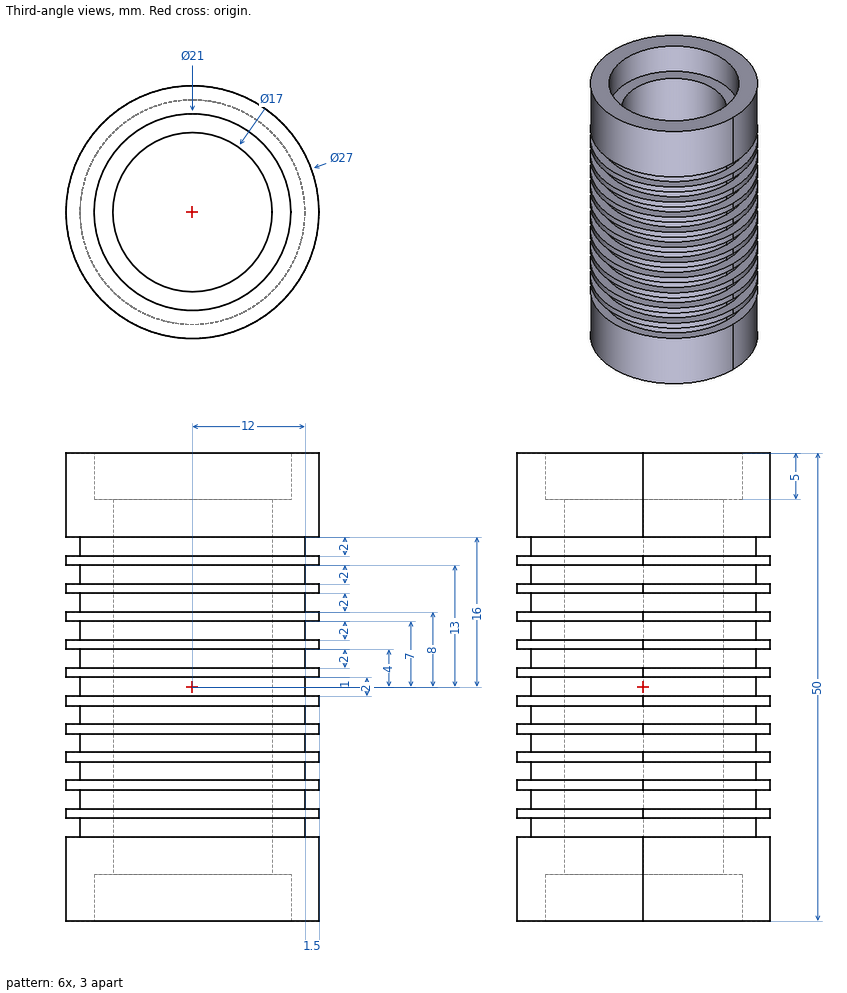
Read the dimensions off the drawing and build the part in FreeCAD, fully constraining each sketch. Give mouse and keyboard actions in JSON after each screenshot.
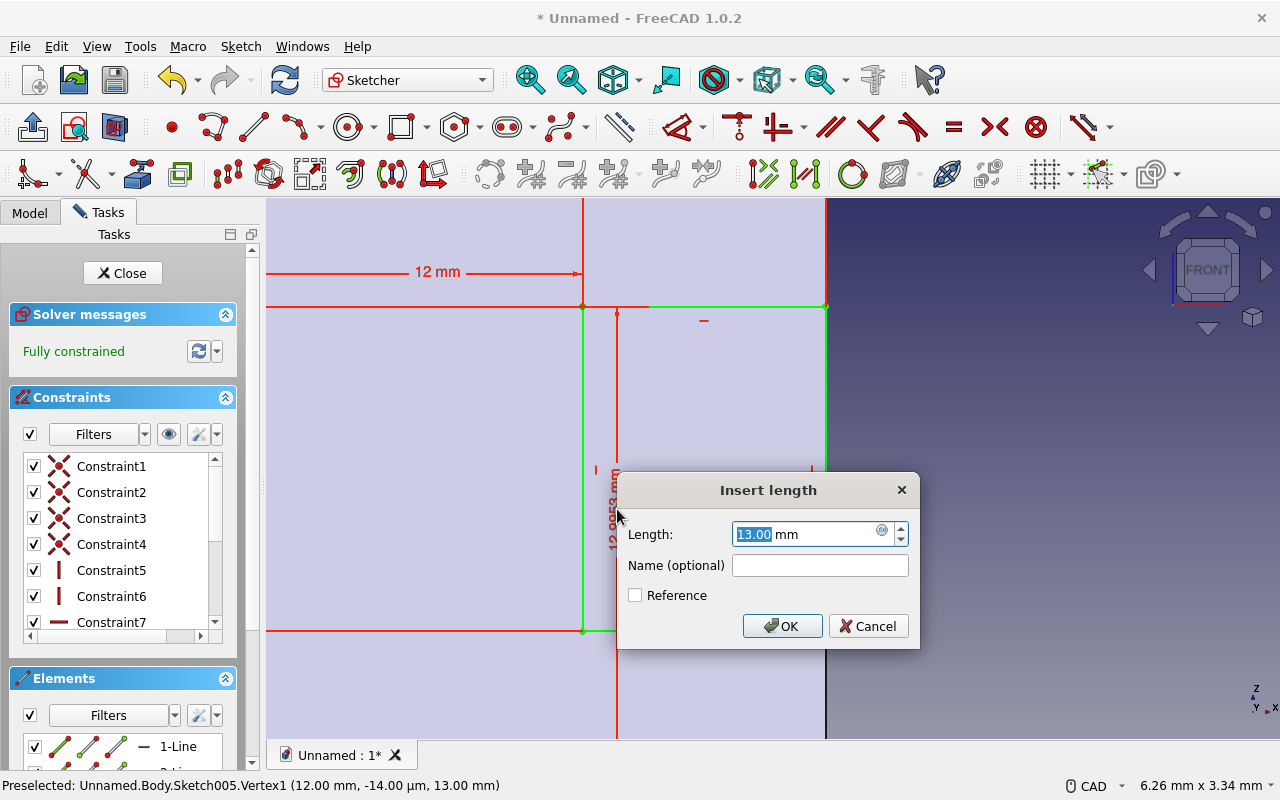
{"action": "type", "text": "13"}
{"action": "key", "text": "Return"}
{"action": "key", "text": "Escape"}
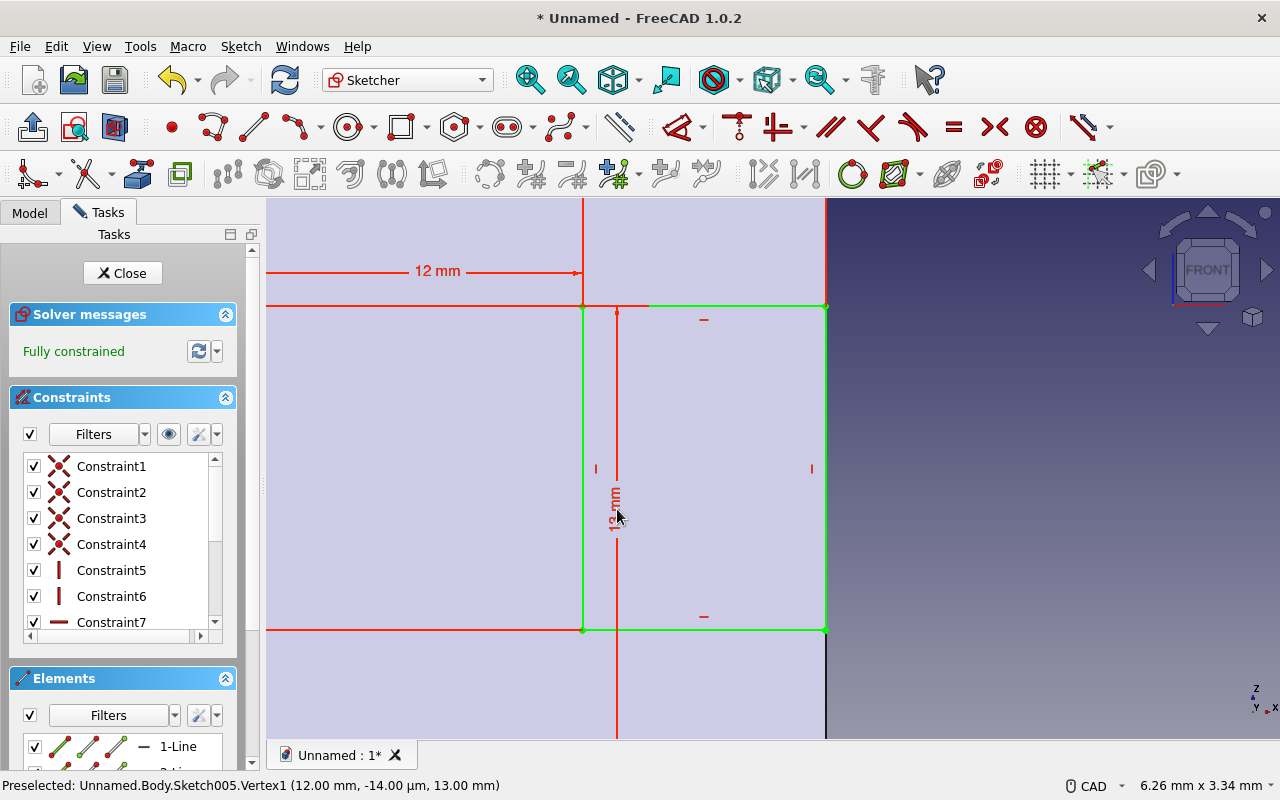
{"action": "left_click", "coordinate": [123, 273]}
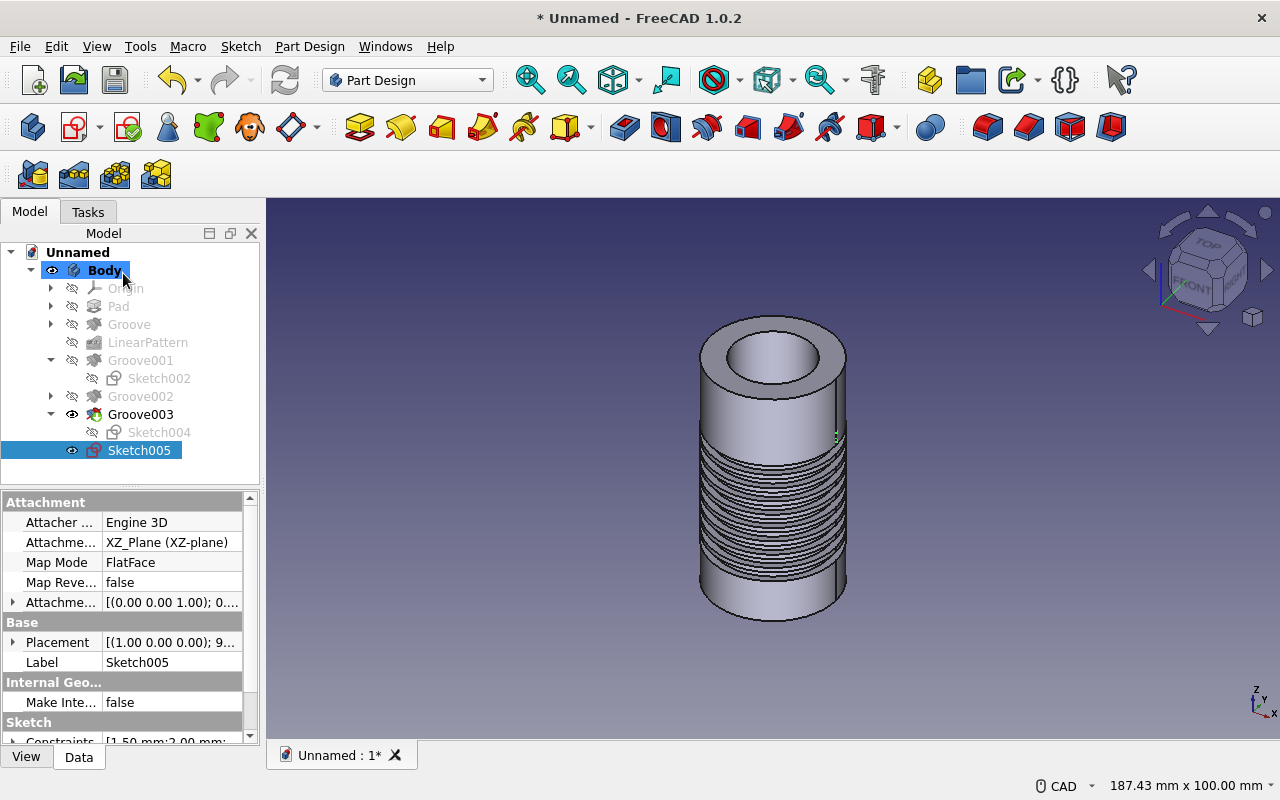
{"action": "left_click", "coordinate": [707, 128]}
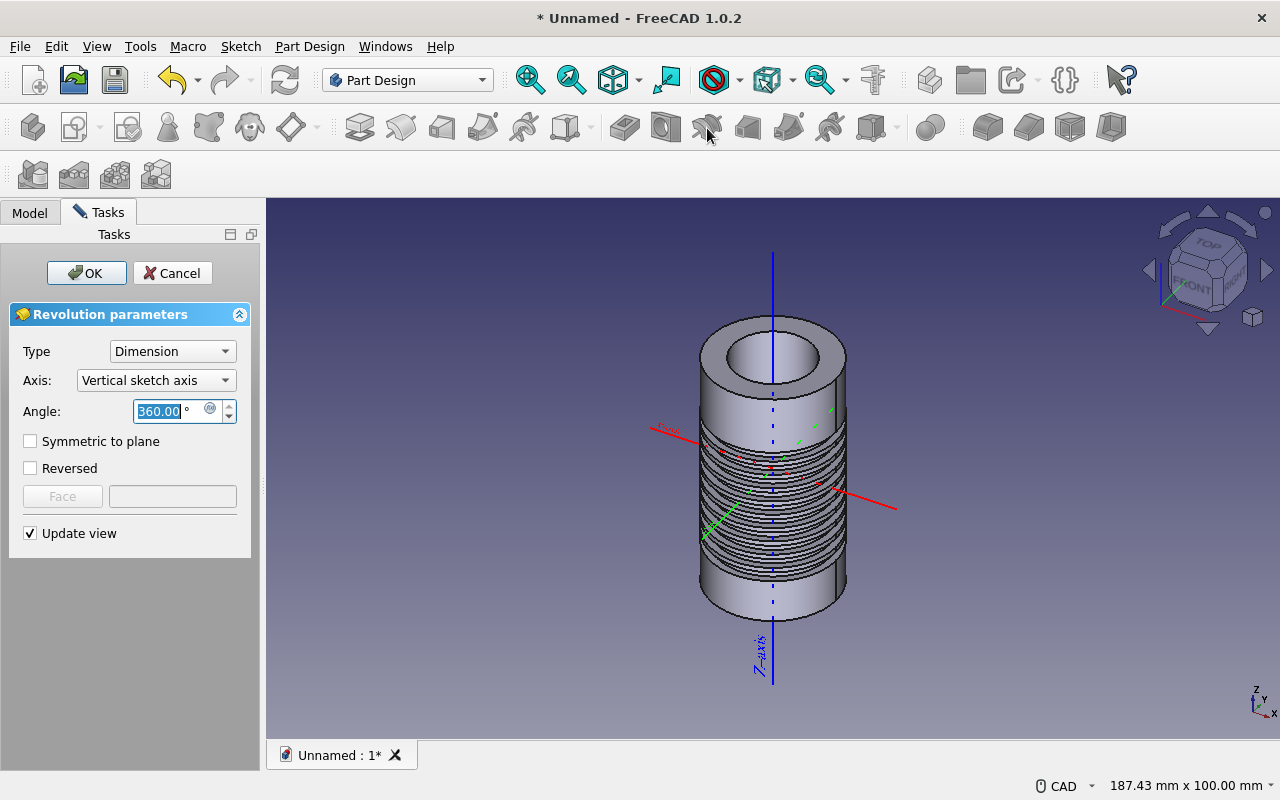
{"action": "left_click", "coordinate": [87, 273]}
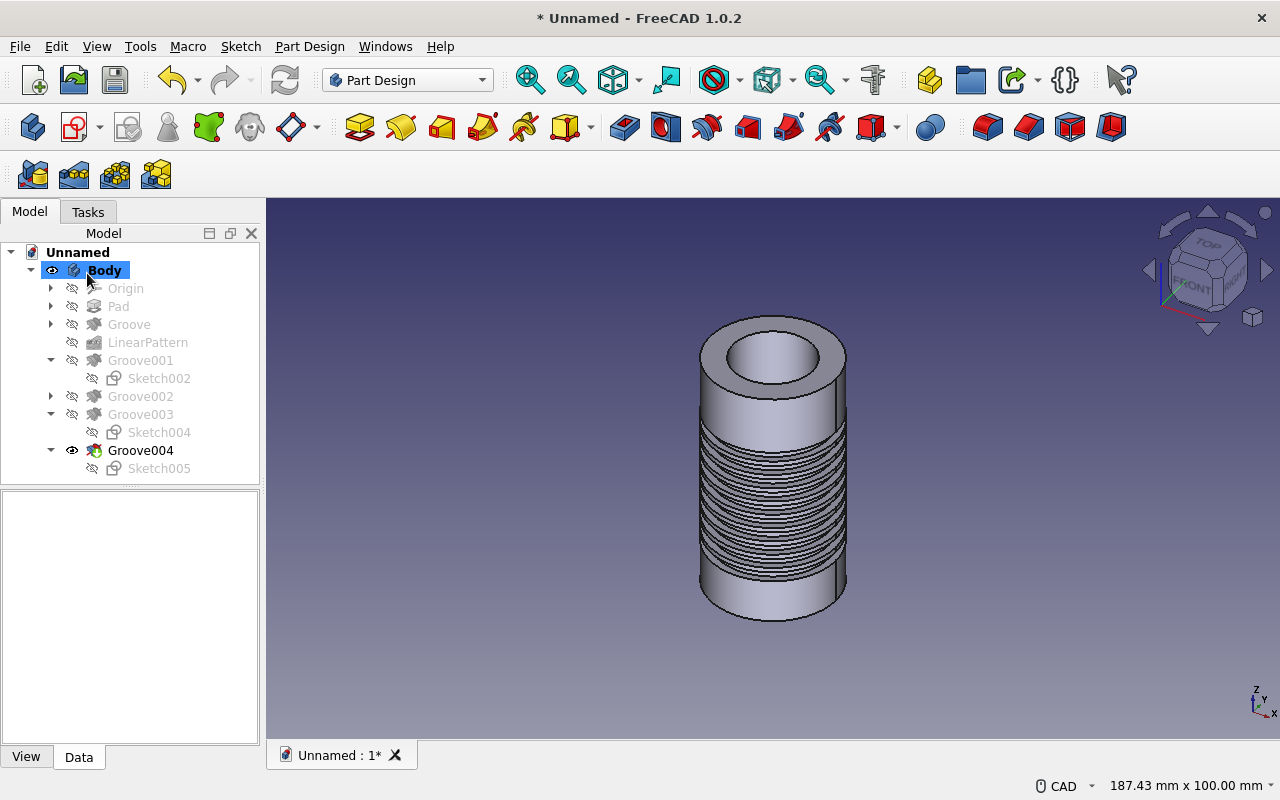
{"action": "left_click", "coordinate": [74, 128]}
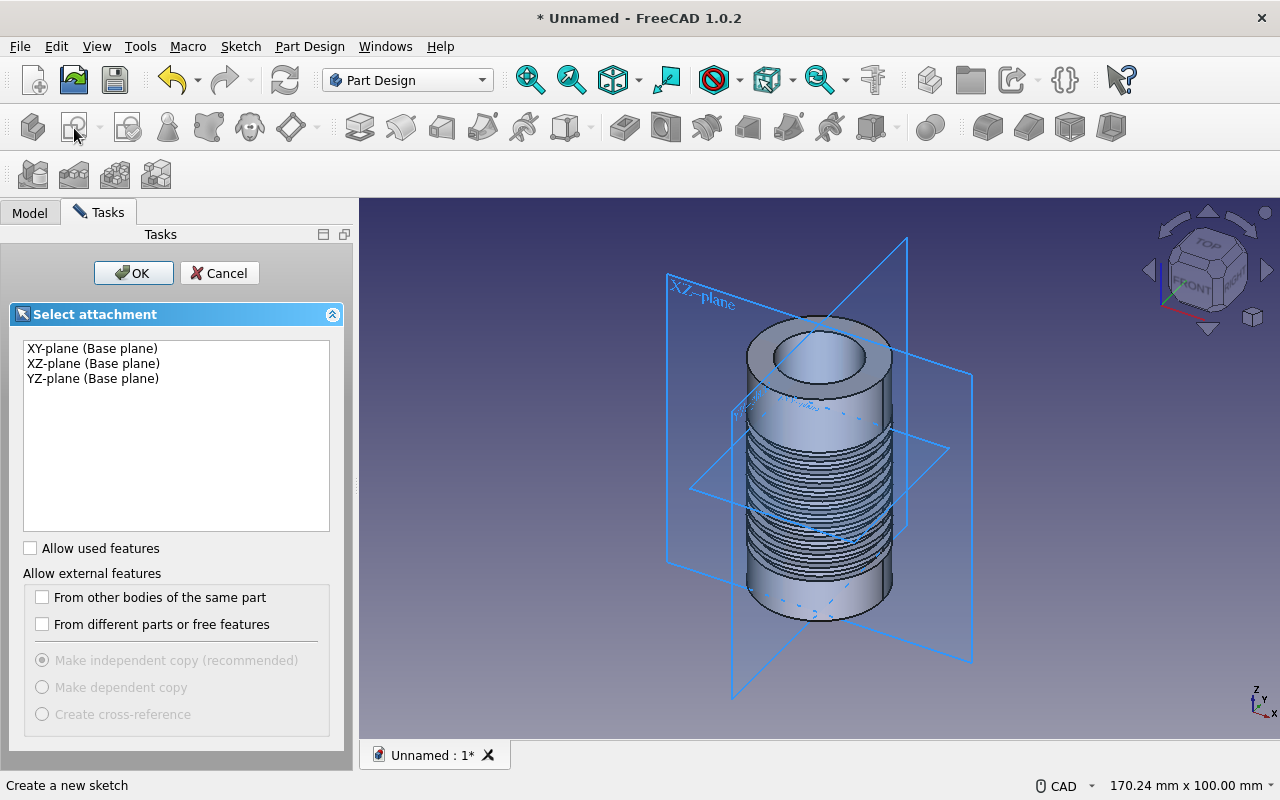
{"action": "left_click", "coordinate": [84, 364]}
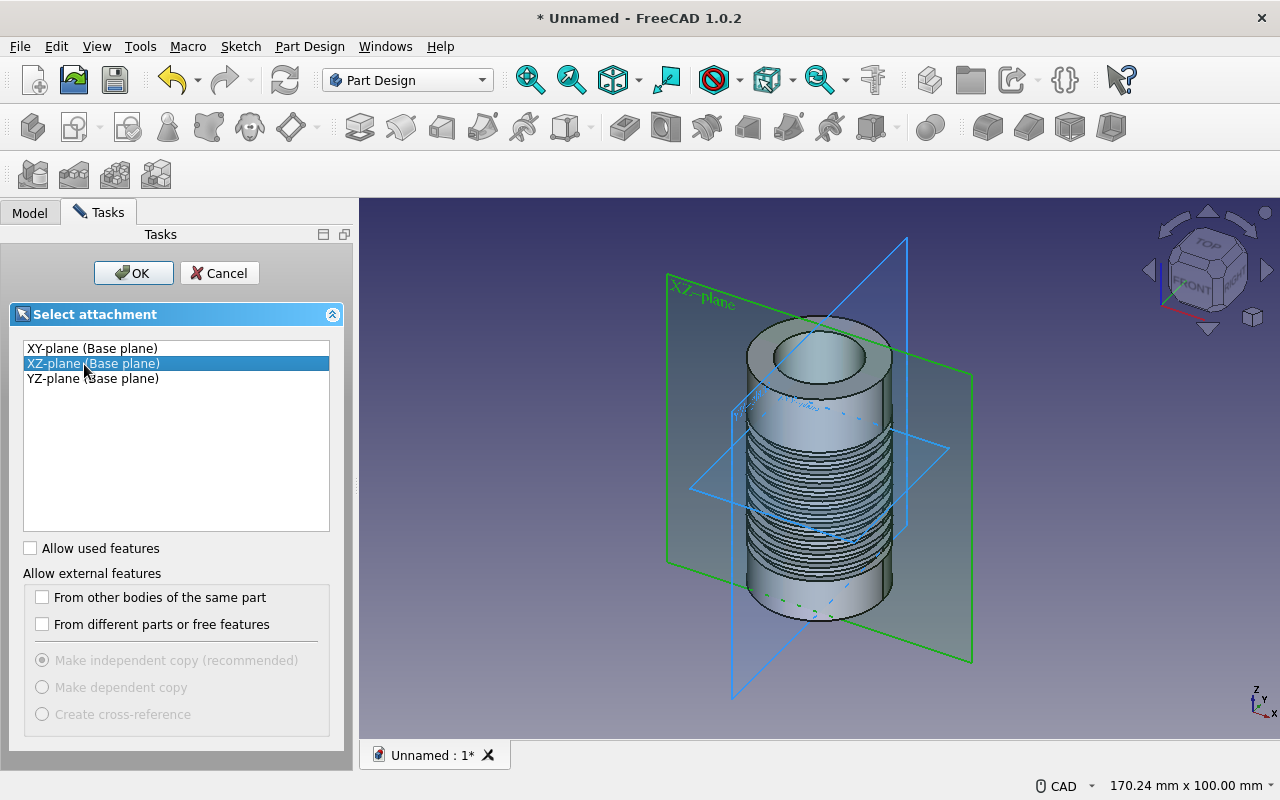
{"action": "left_click", "coordinate": [134, 273]}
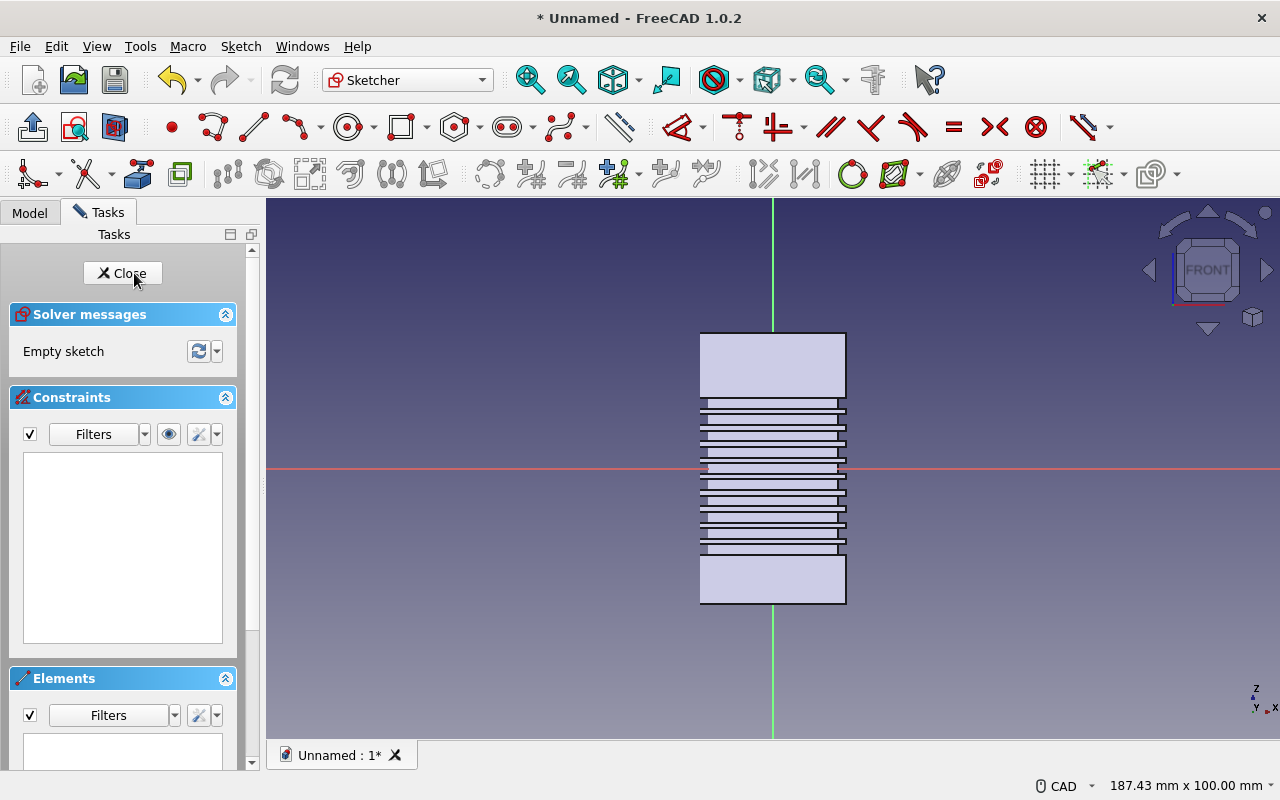
{"action": "left_click", "coordinate": [115, 128]}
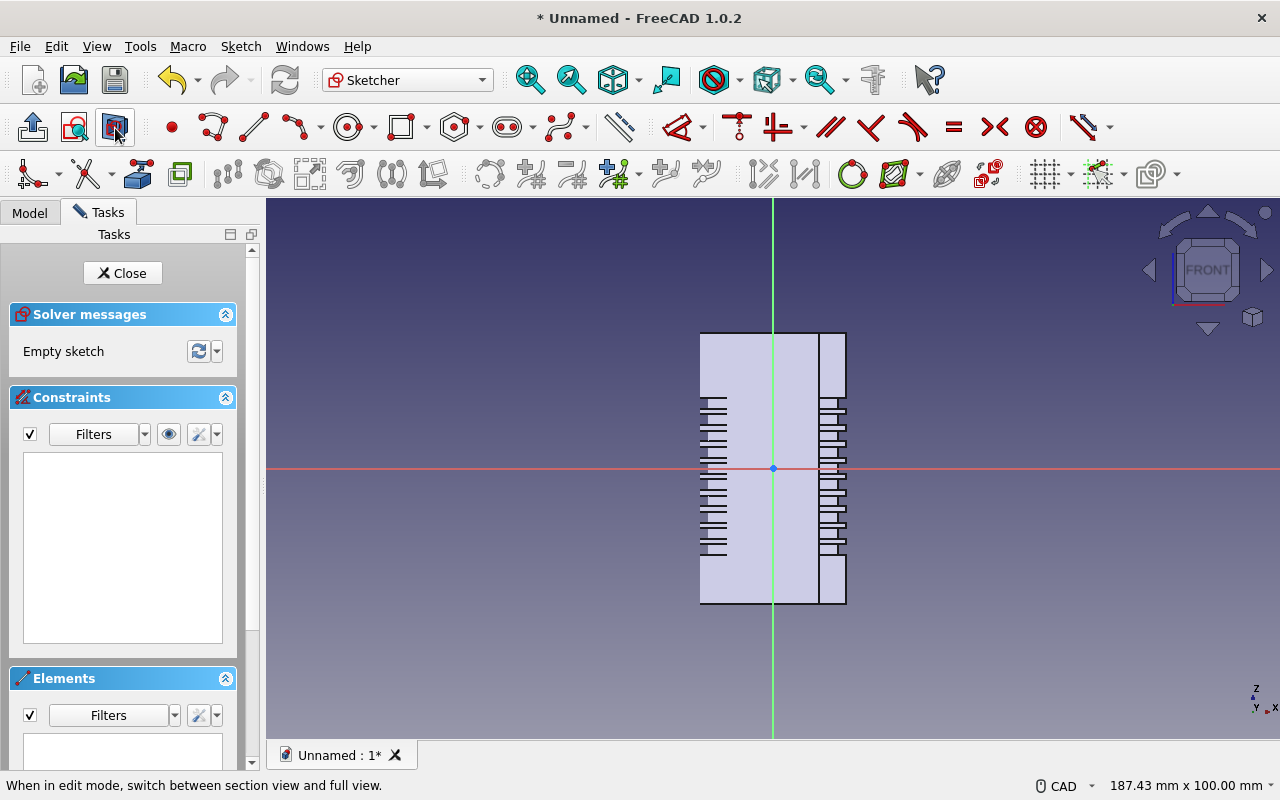
{"action": "scroll", "coordinate": [849, 383], "scroll_direction": "up", "scroll_amount": 15}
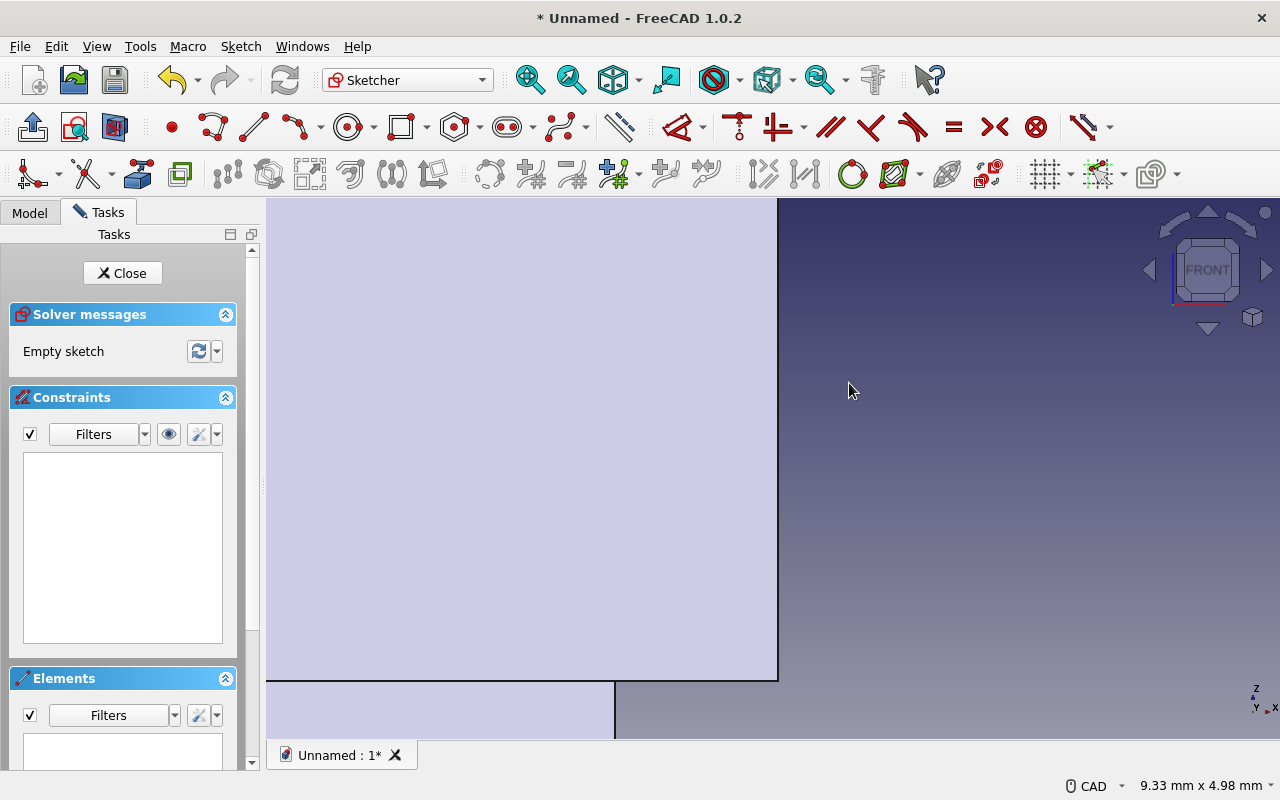
{"action": "scroll", "coordinate": [682, 454], "scroll_direction": "up", "scroll_amount": 2}